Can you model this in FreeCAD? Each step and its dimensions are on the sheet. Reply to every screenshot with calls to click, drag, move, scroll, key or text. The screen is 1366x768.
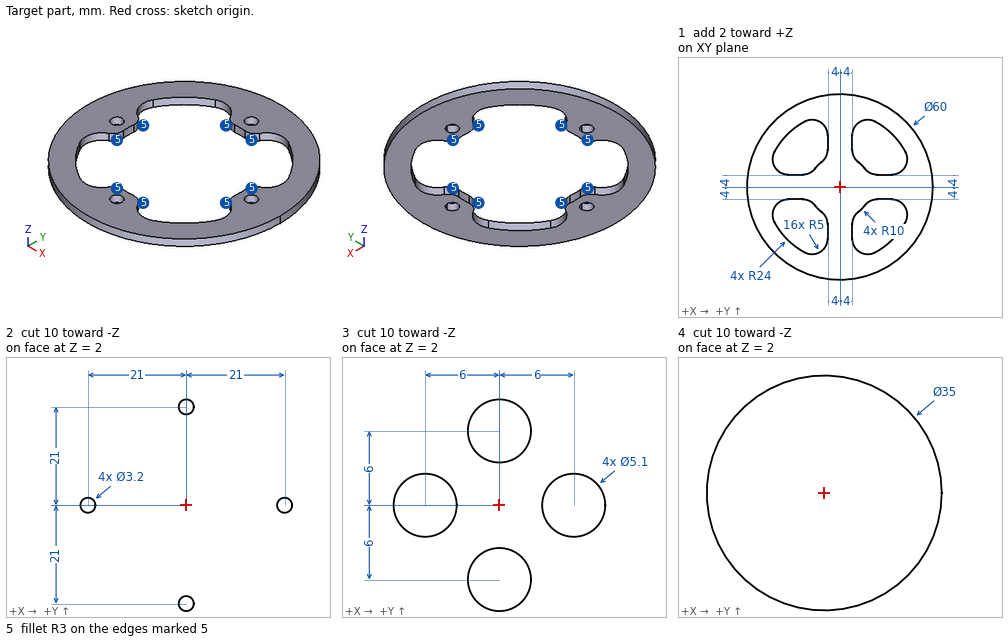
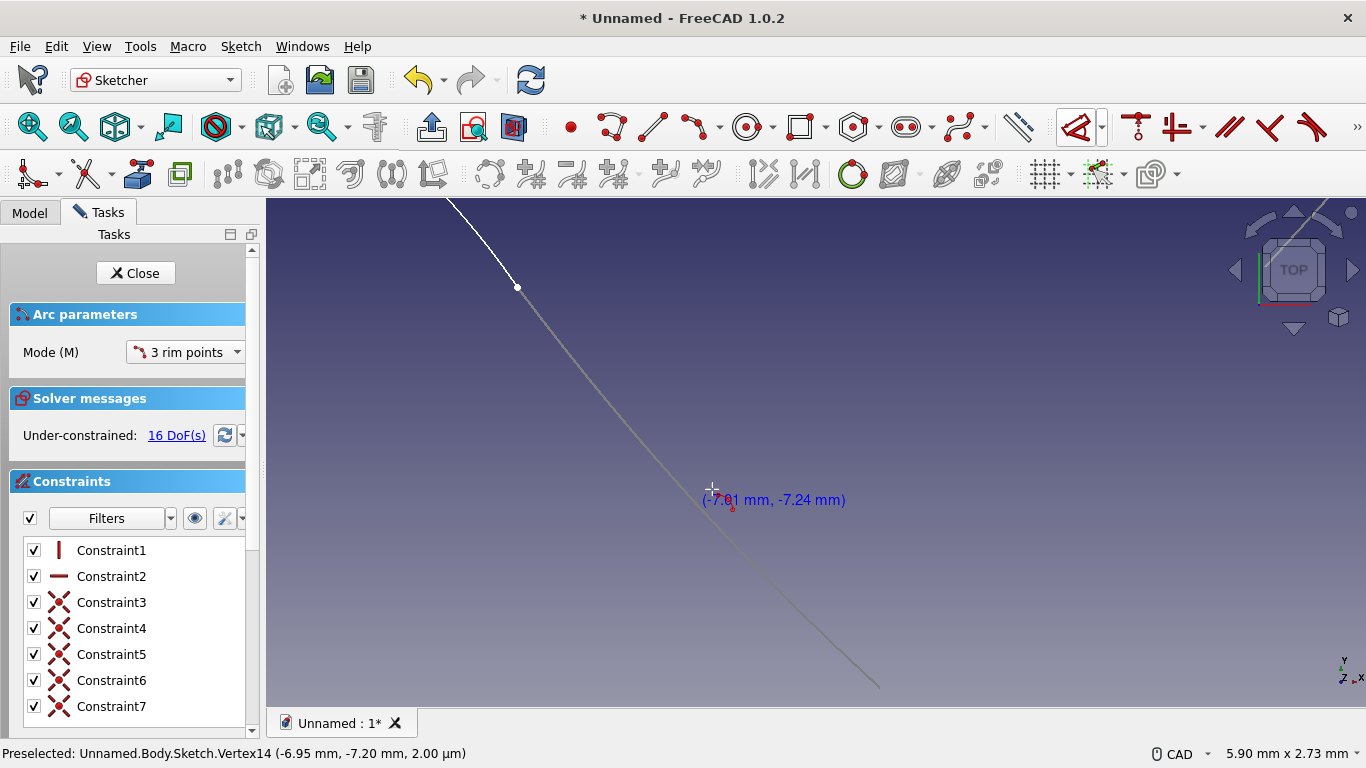
click(685, 473)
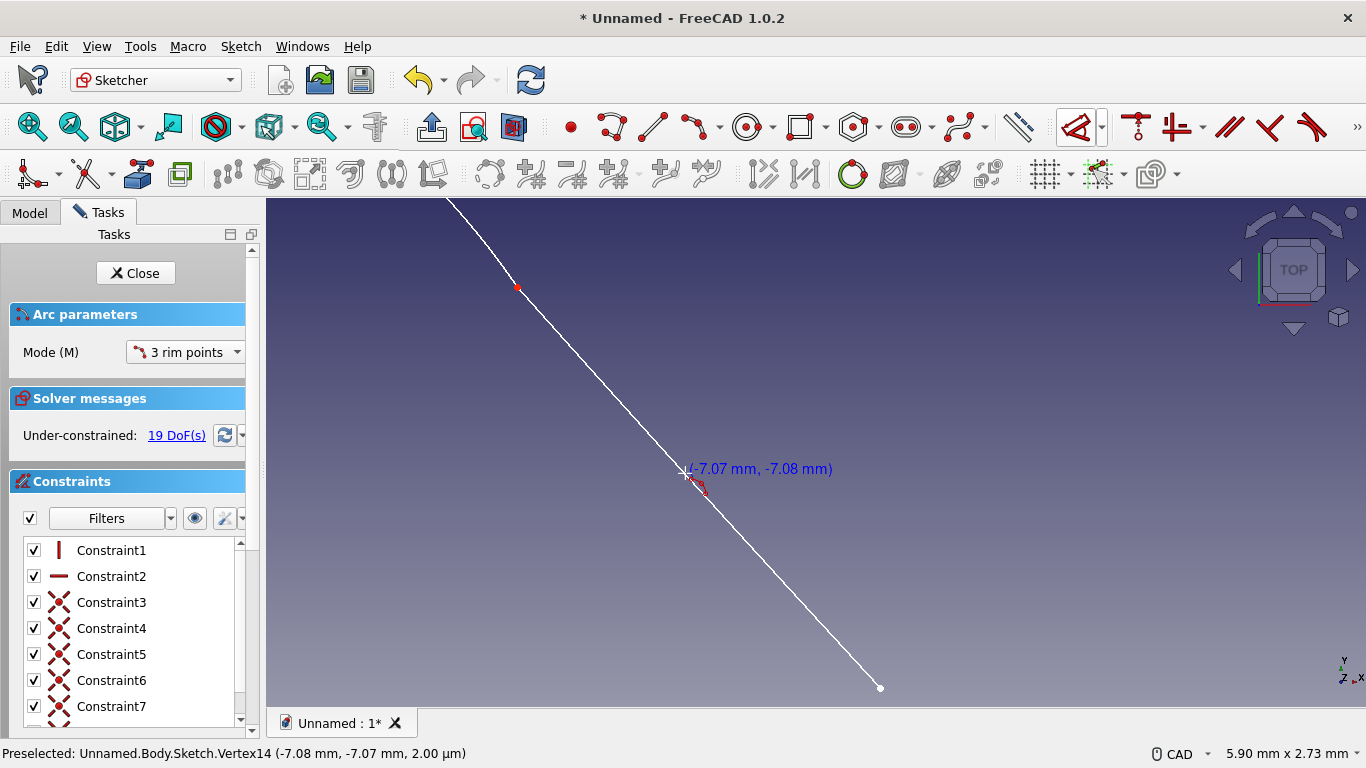
scroll(704, 497, down, 17)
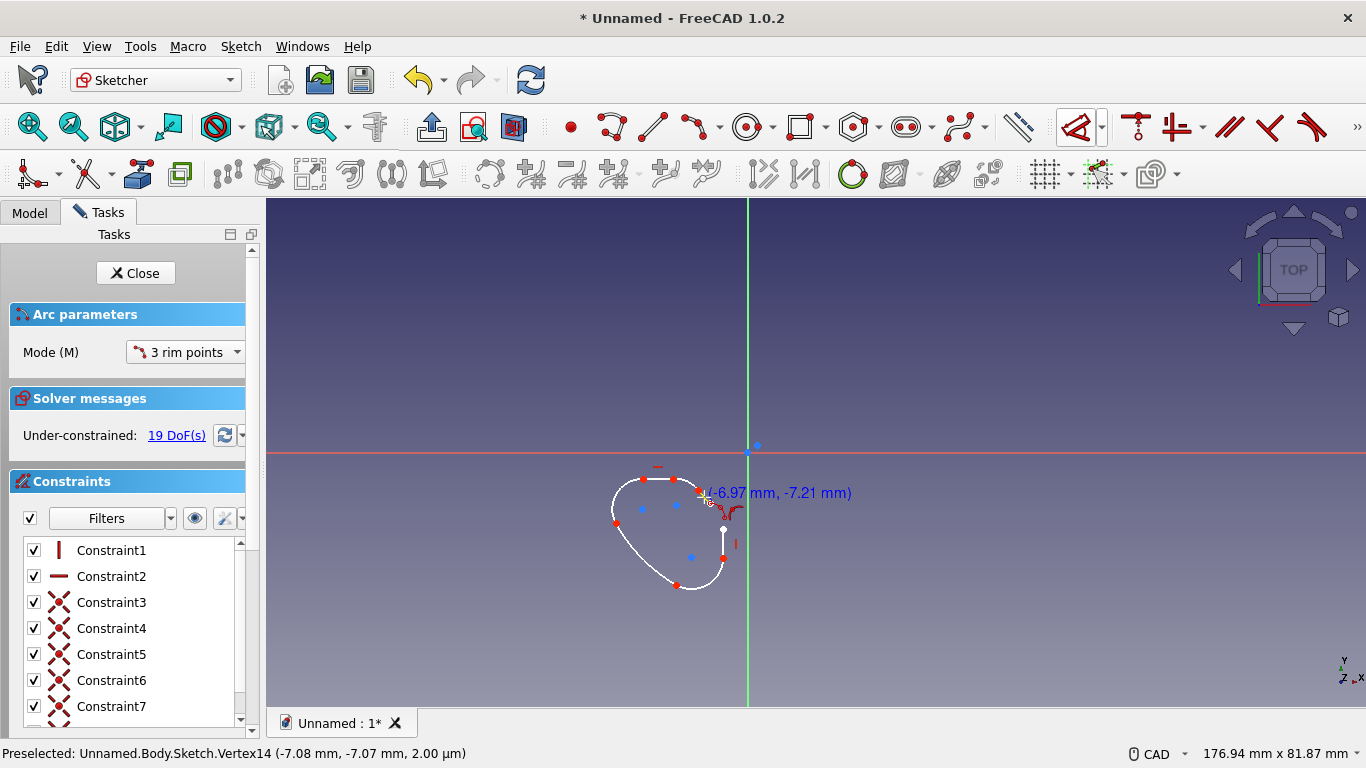
click(710, 504)
click(723, 529)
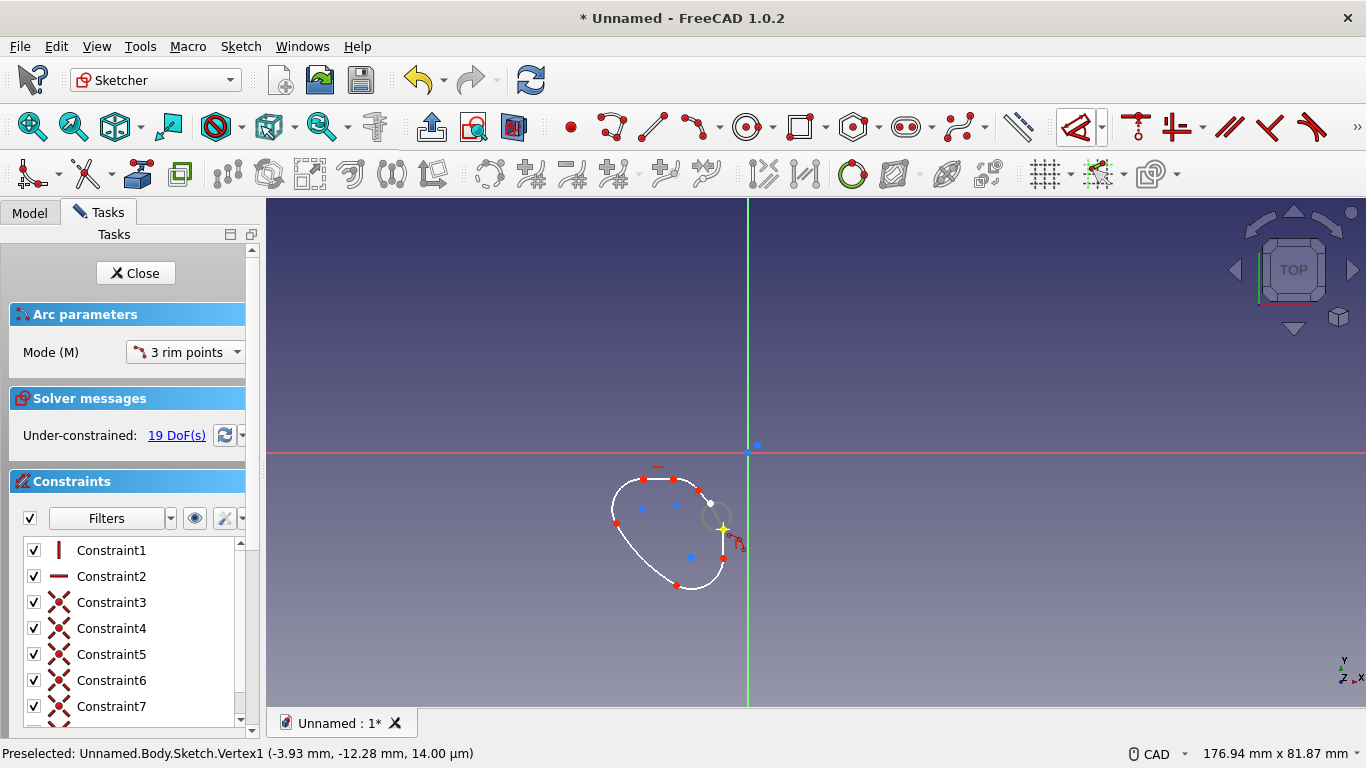
scroll(720, 514, up, 8)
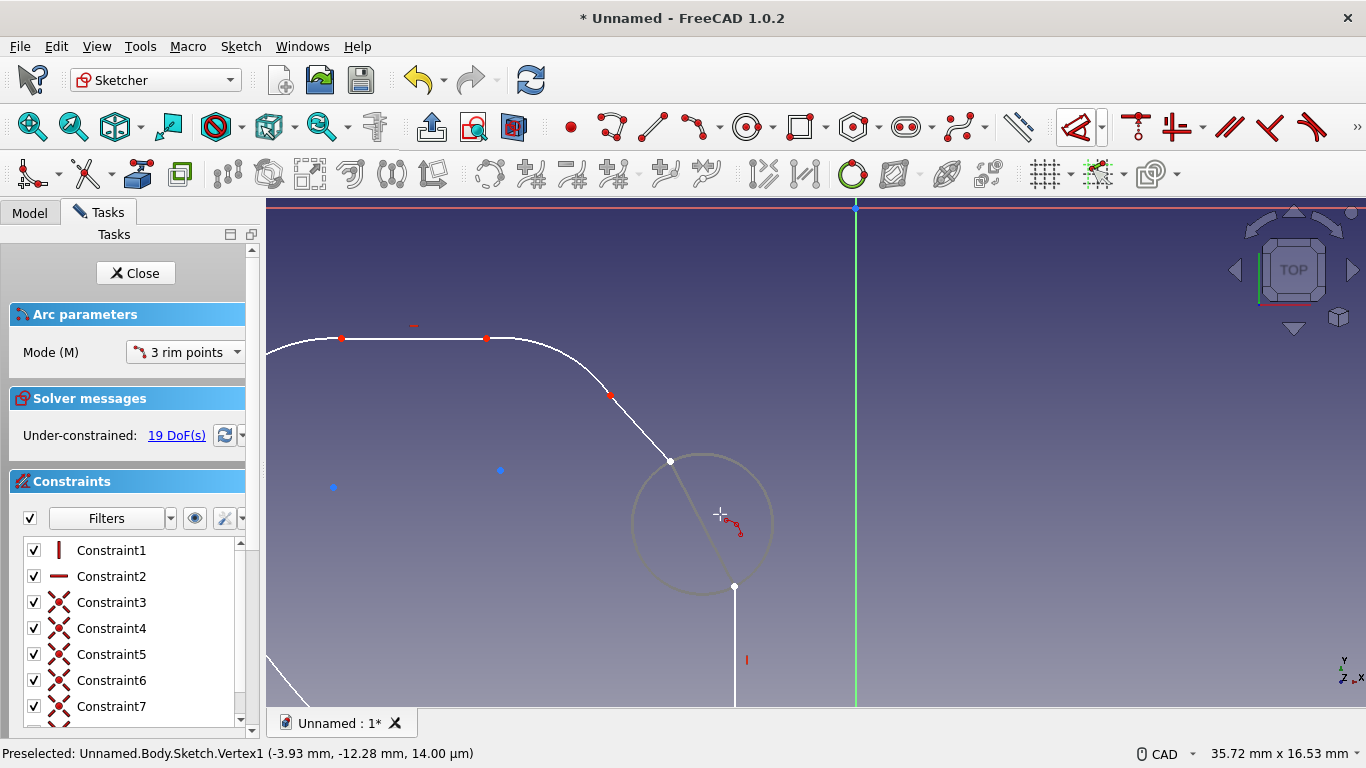
click(716, 509)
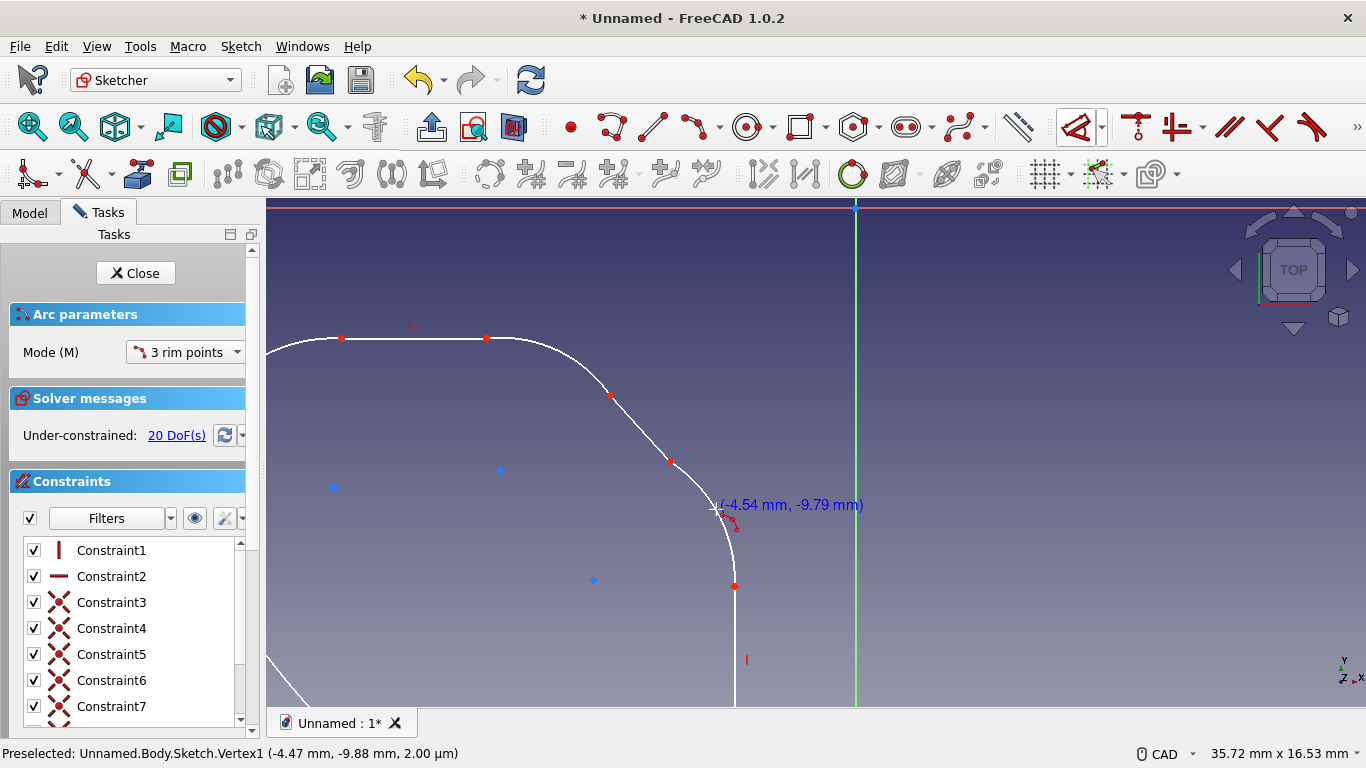
key(g)
key(l)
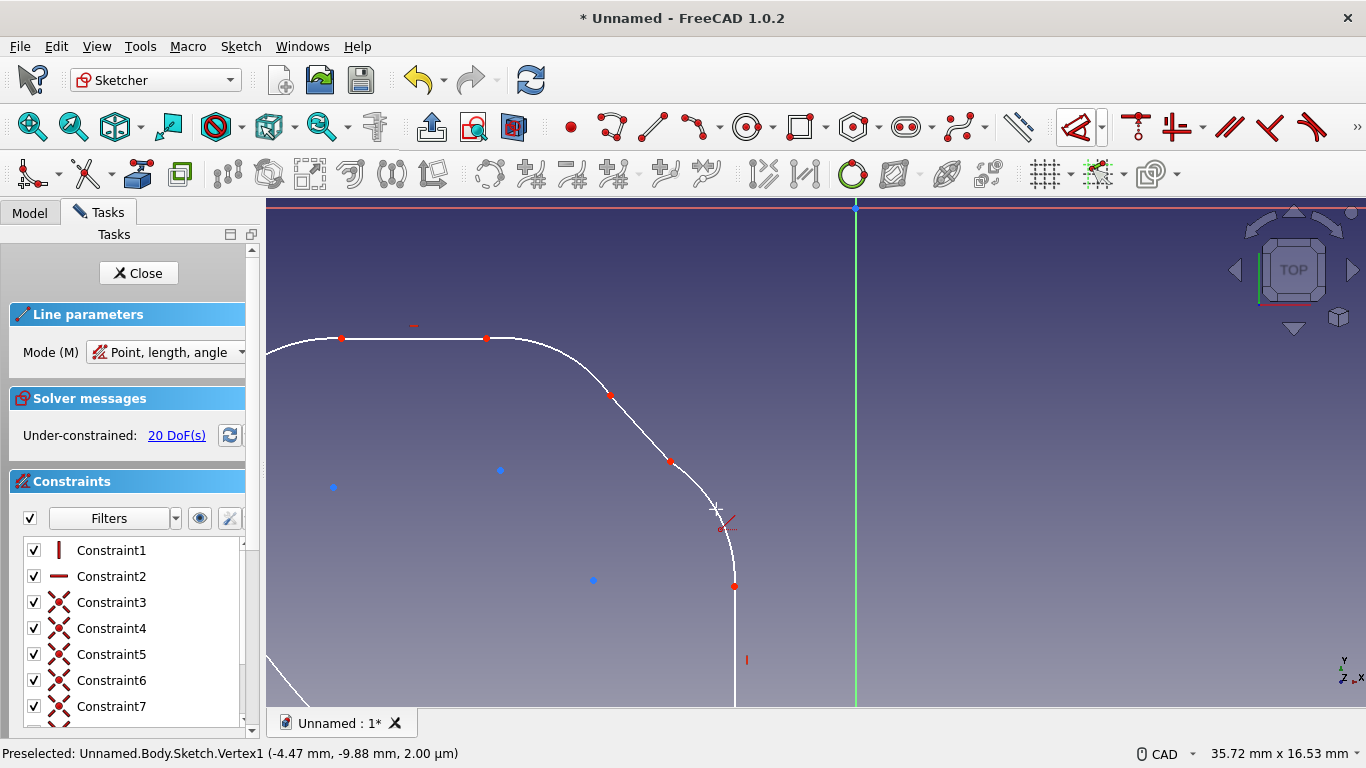
scroll(726, 501, down, 9)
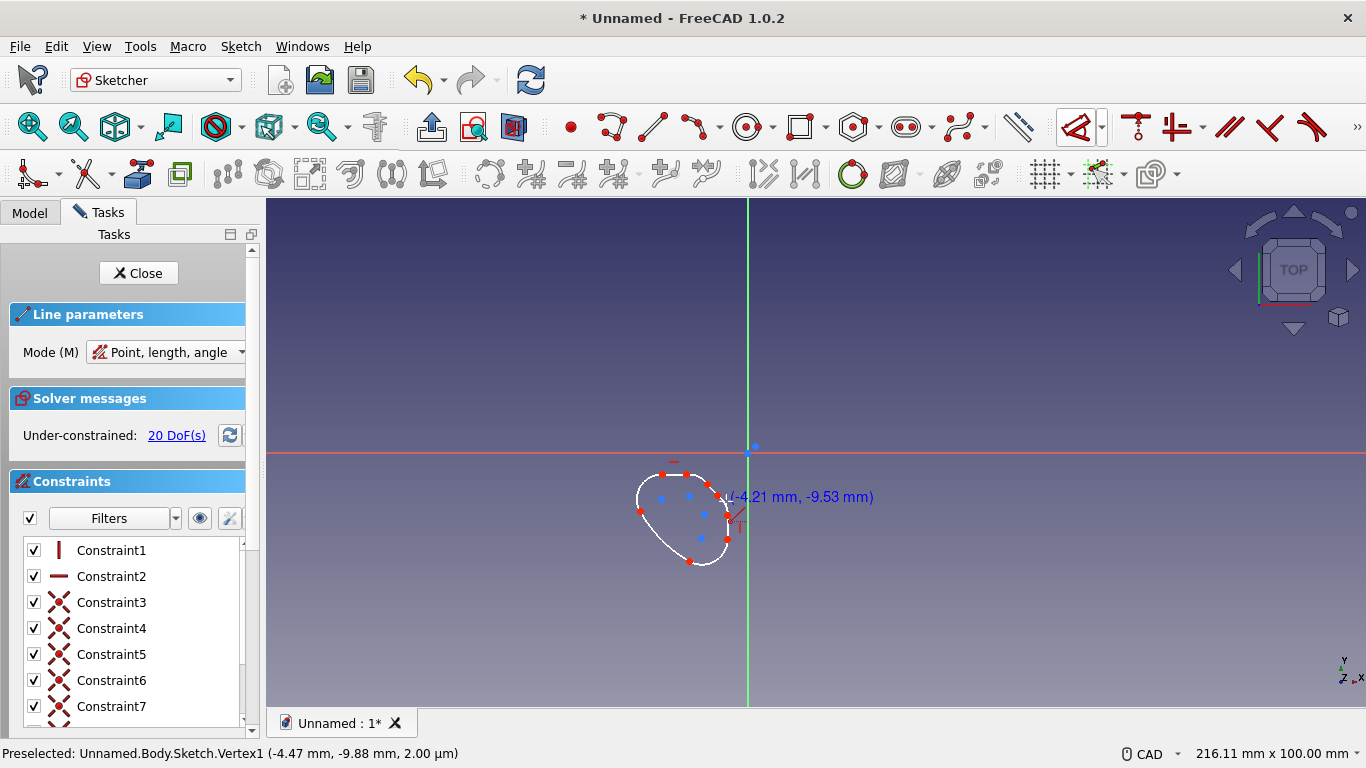
click(809, 473)
click(833, 473)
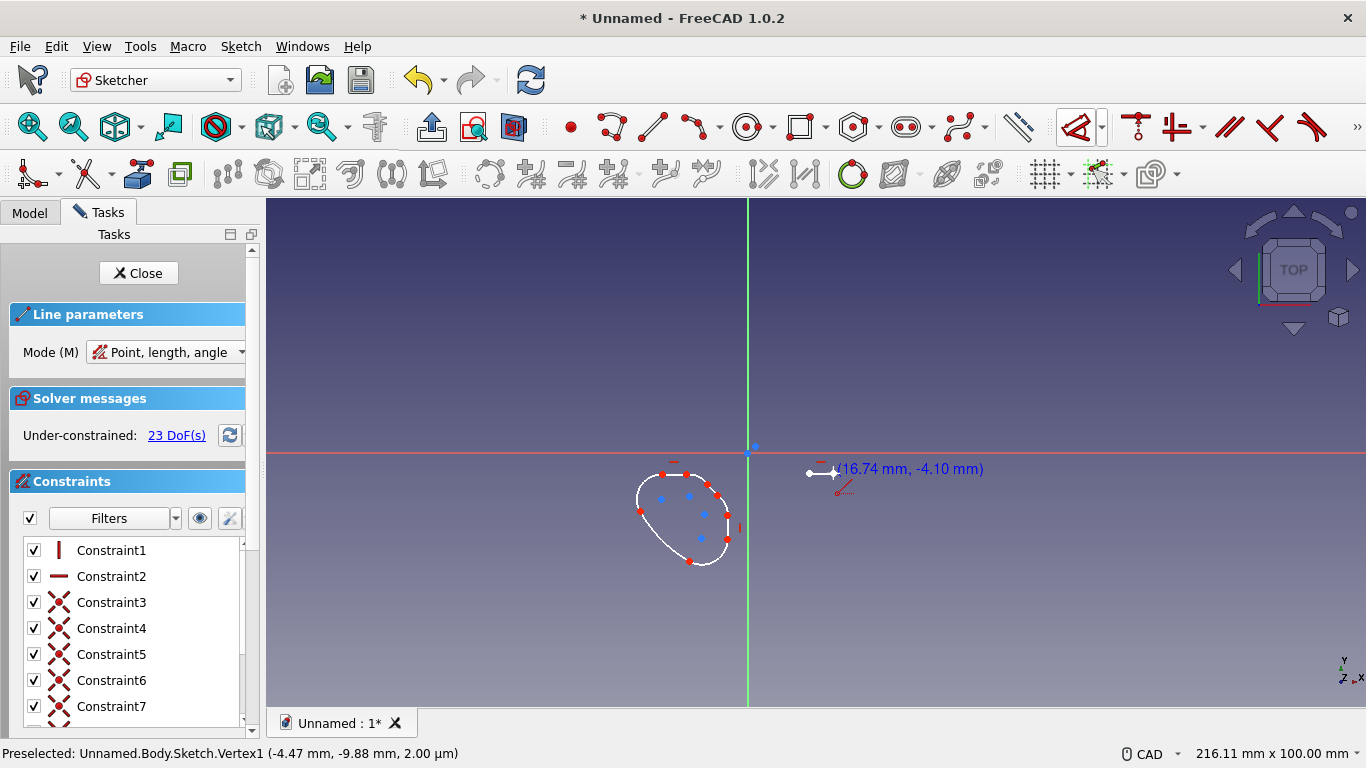
click(768, 538)
click(768, 514)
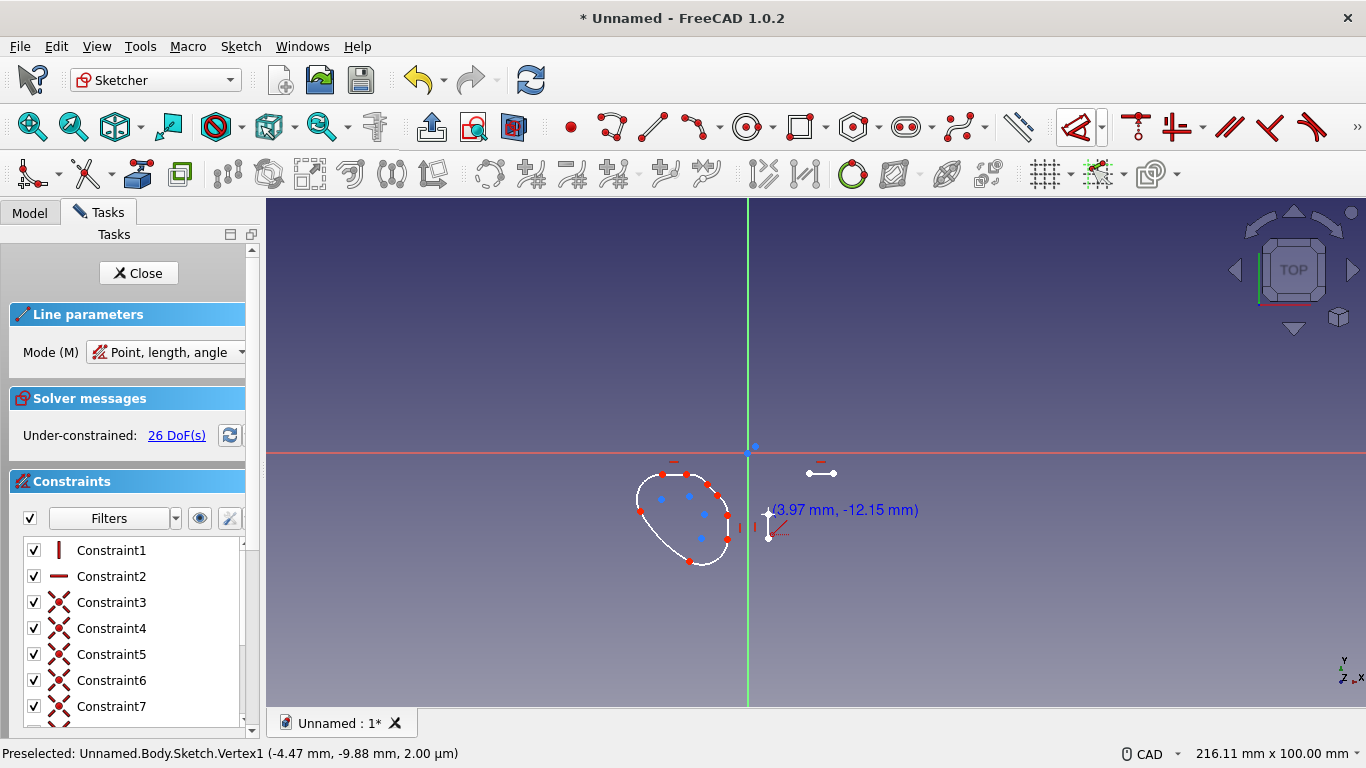
click(694, 128)